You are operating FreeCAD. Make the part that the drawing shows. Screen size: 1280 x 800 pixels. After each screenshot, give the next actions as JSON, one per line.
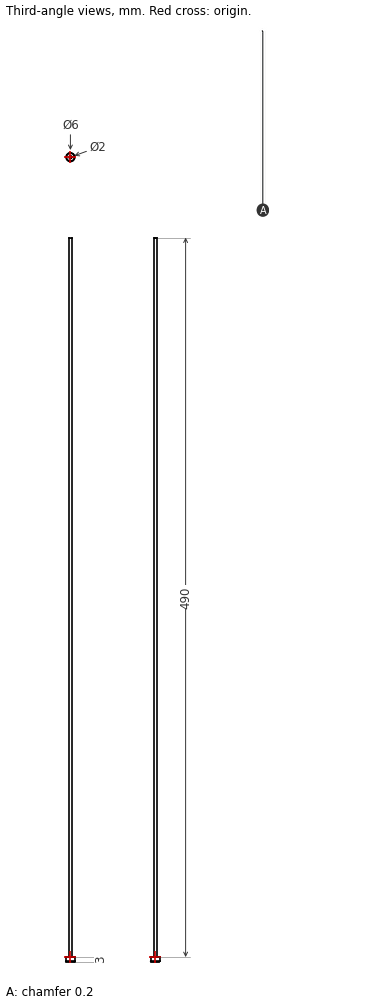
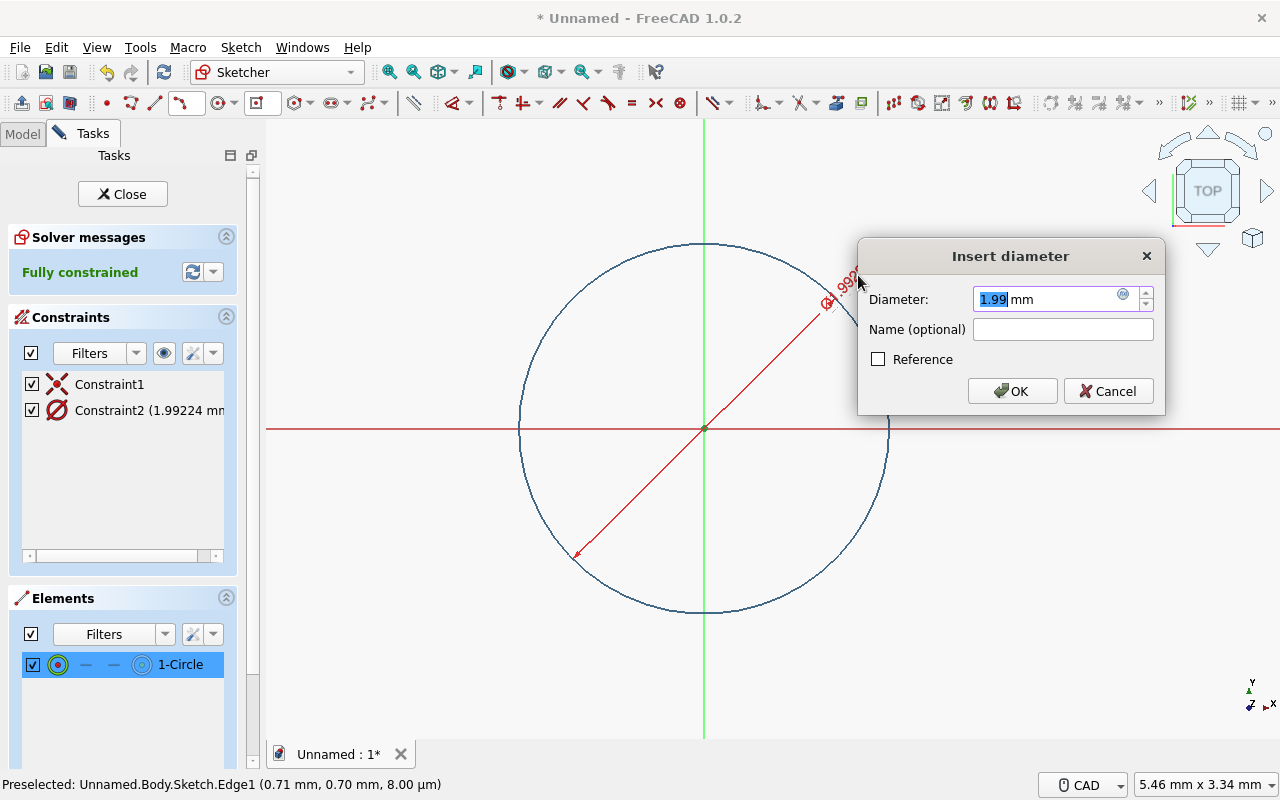
{"action": "type", "text": "2"}
{"action": "key", "text": "Return"}
{"action": "key", "text": "Escape"}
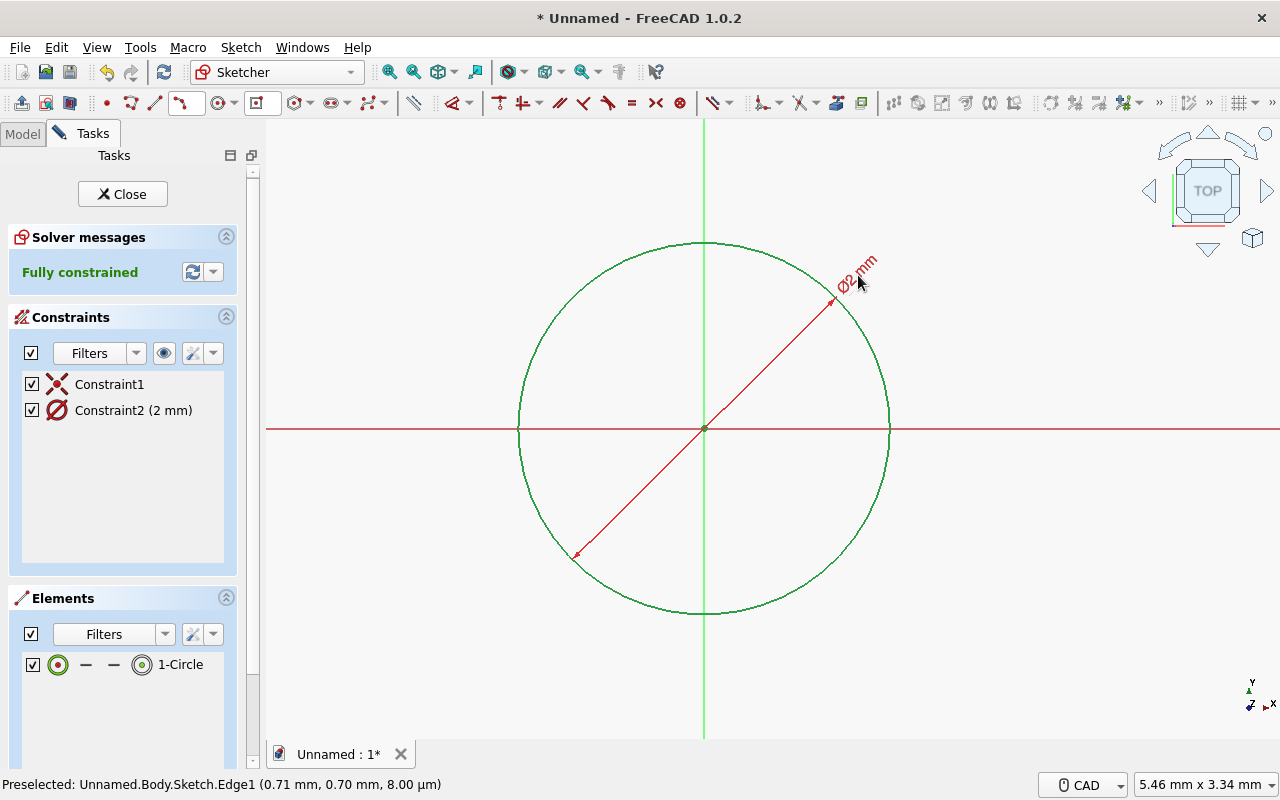
{"action": "left_click", "coordinate": [123, 194]}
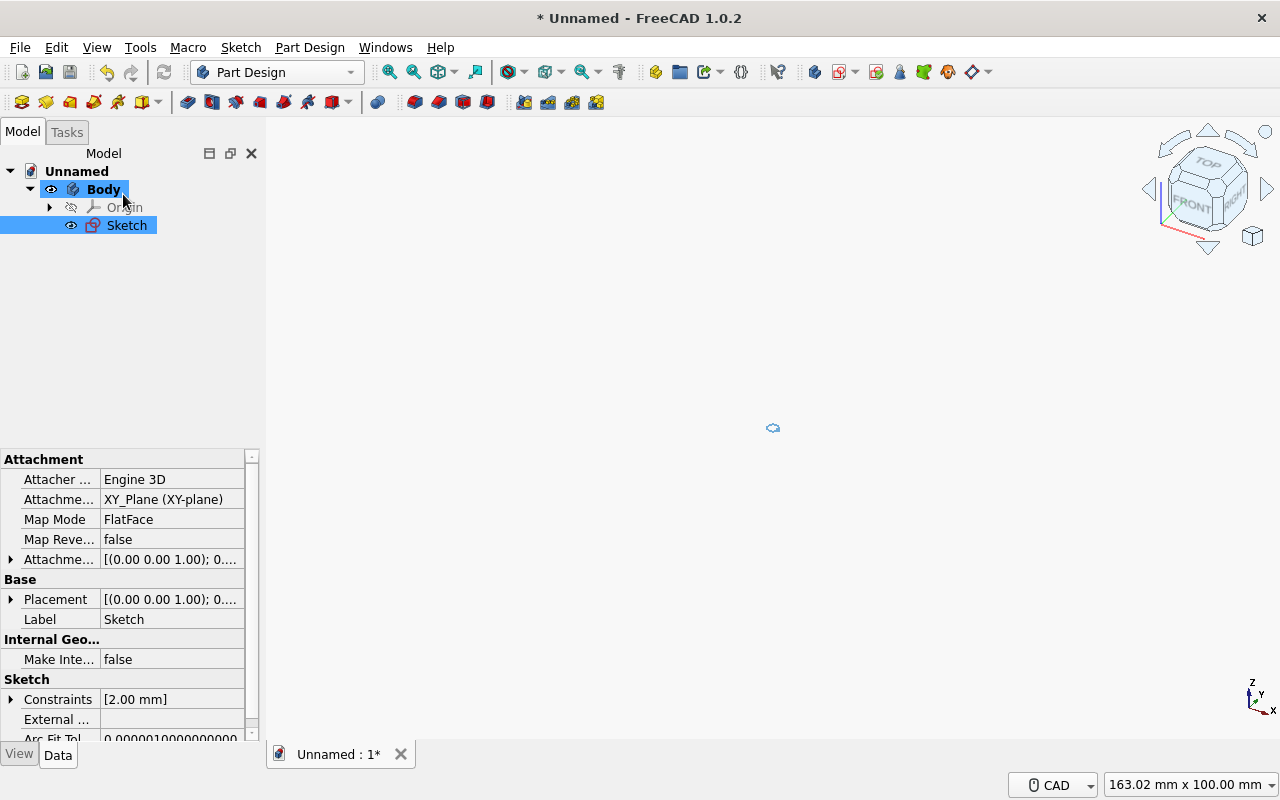
{"action": "left_click", "coordinate": [22, 102]}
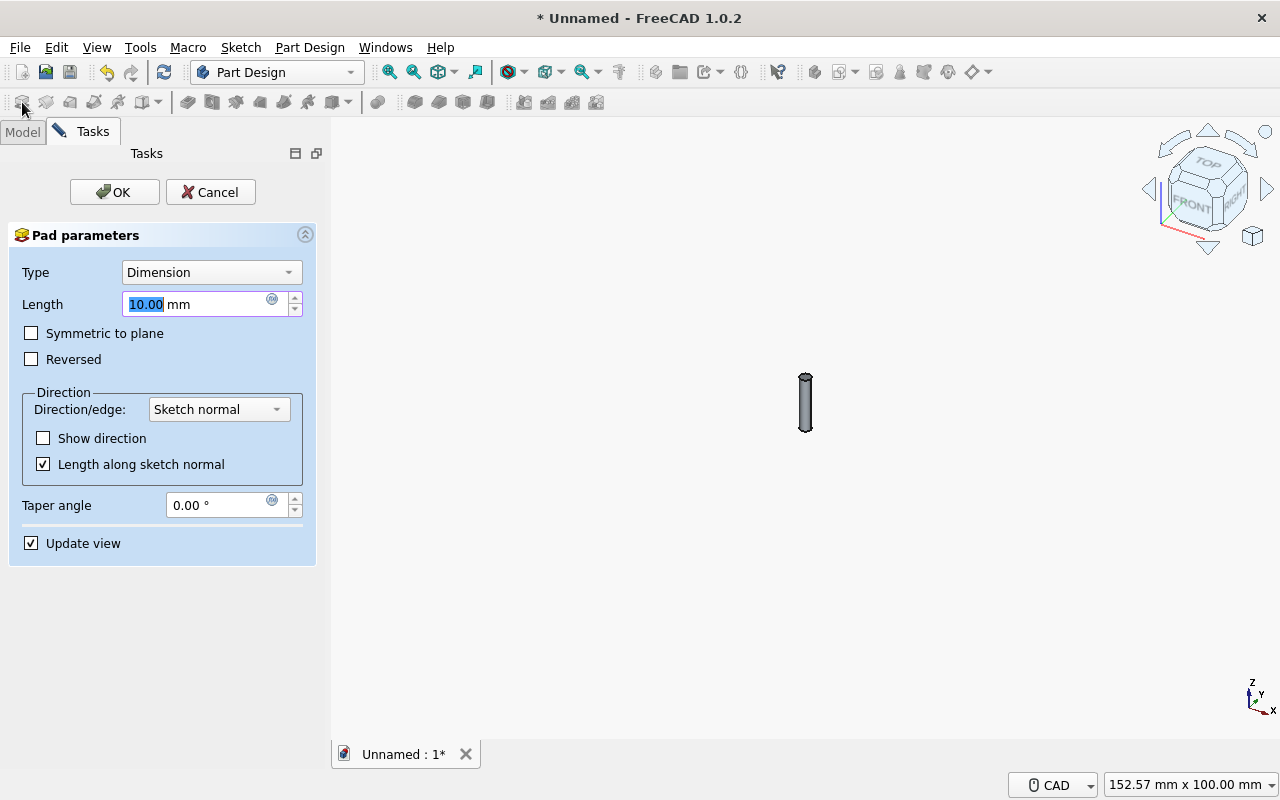
{"action": "type", "text": "490"}
{"action": "key", "text": "Tab"}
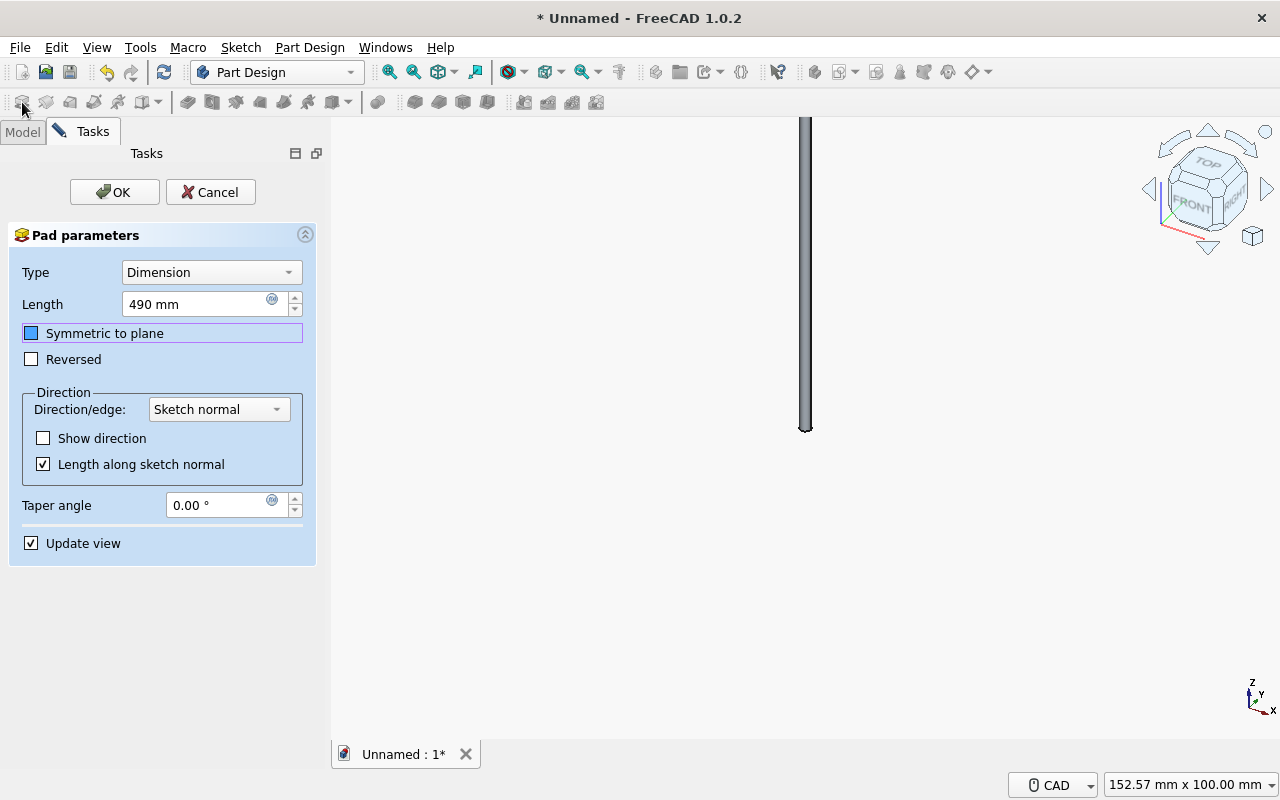
{"action": "left_click", "coordinate": [115, 192]}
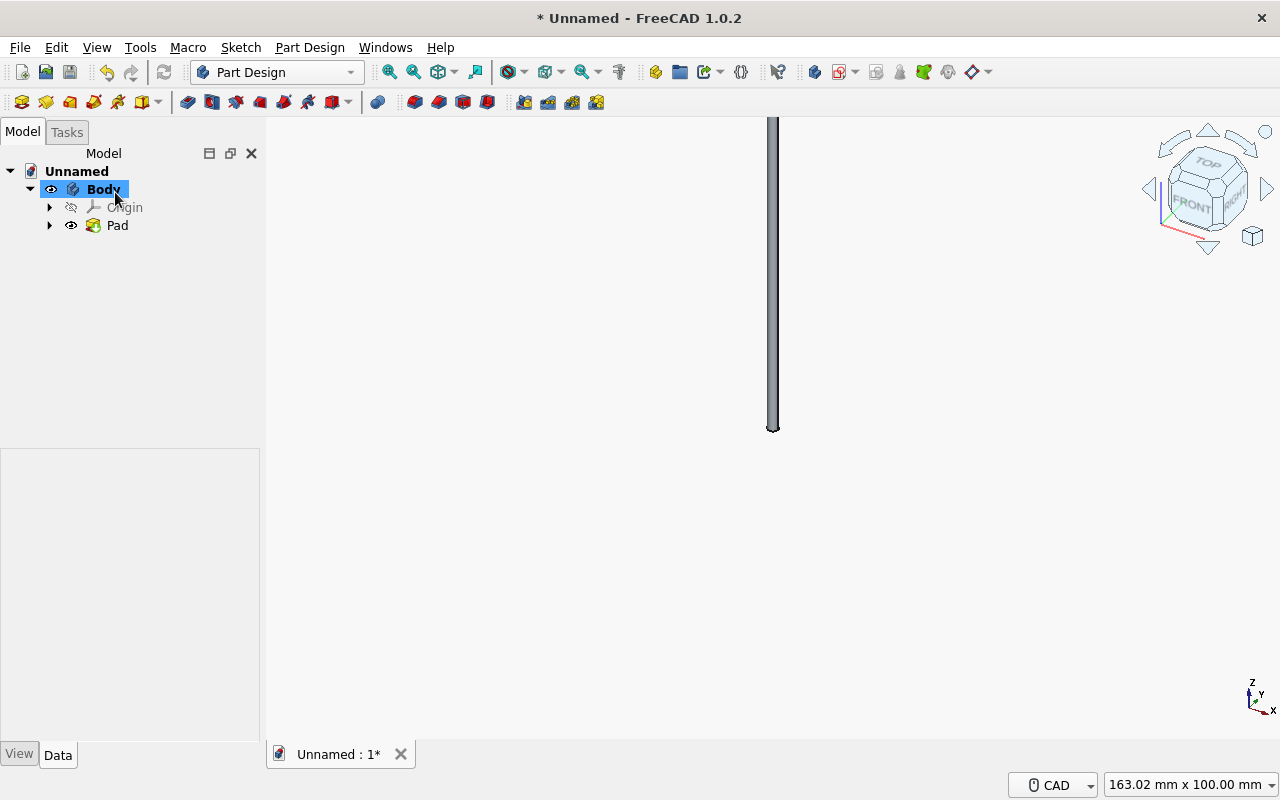
{"action": "key", "text": "v f"}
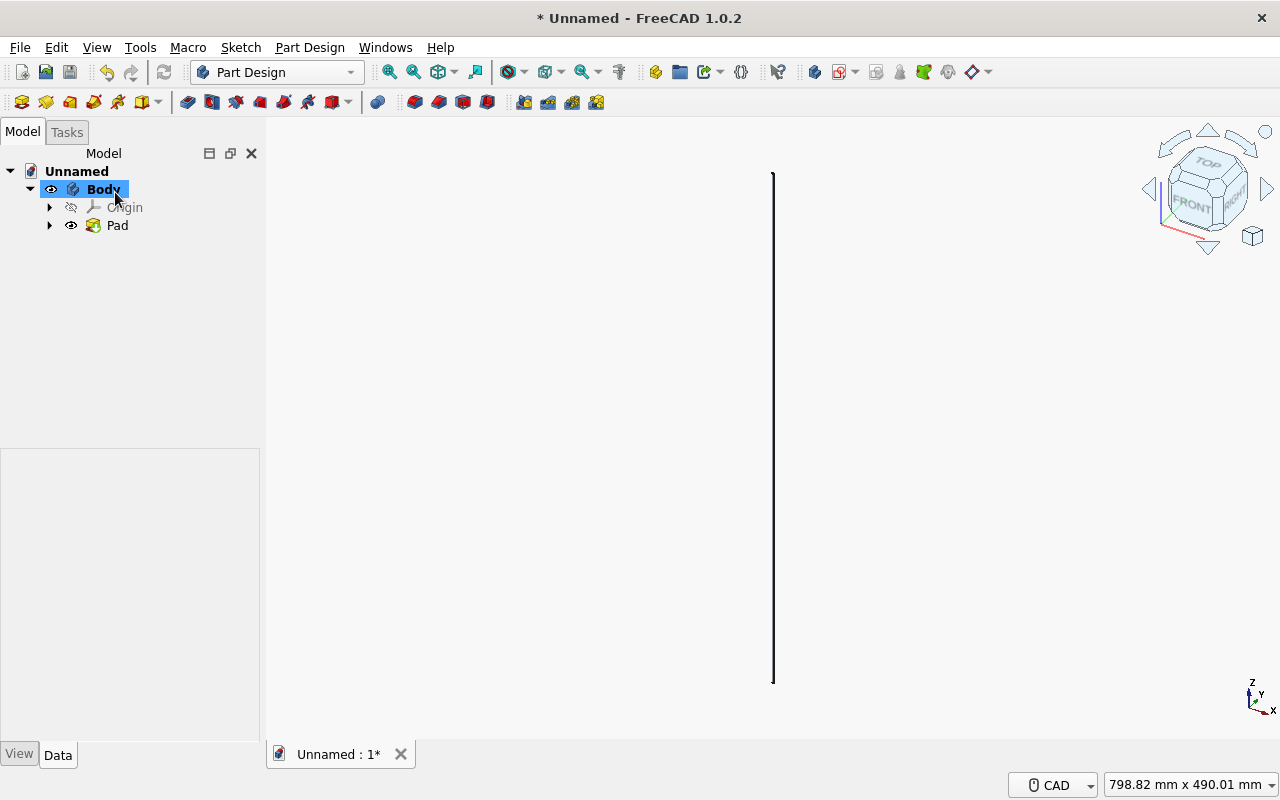
{"action": "key", "text": "5"}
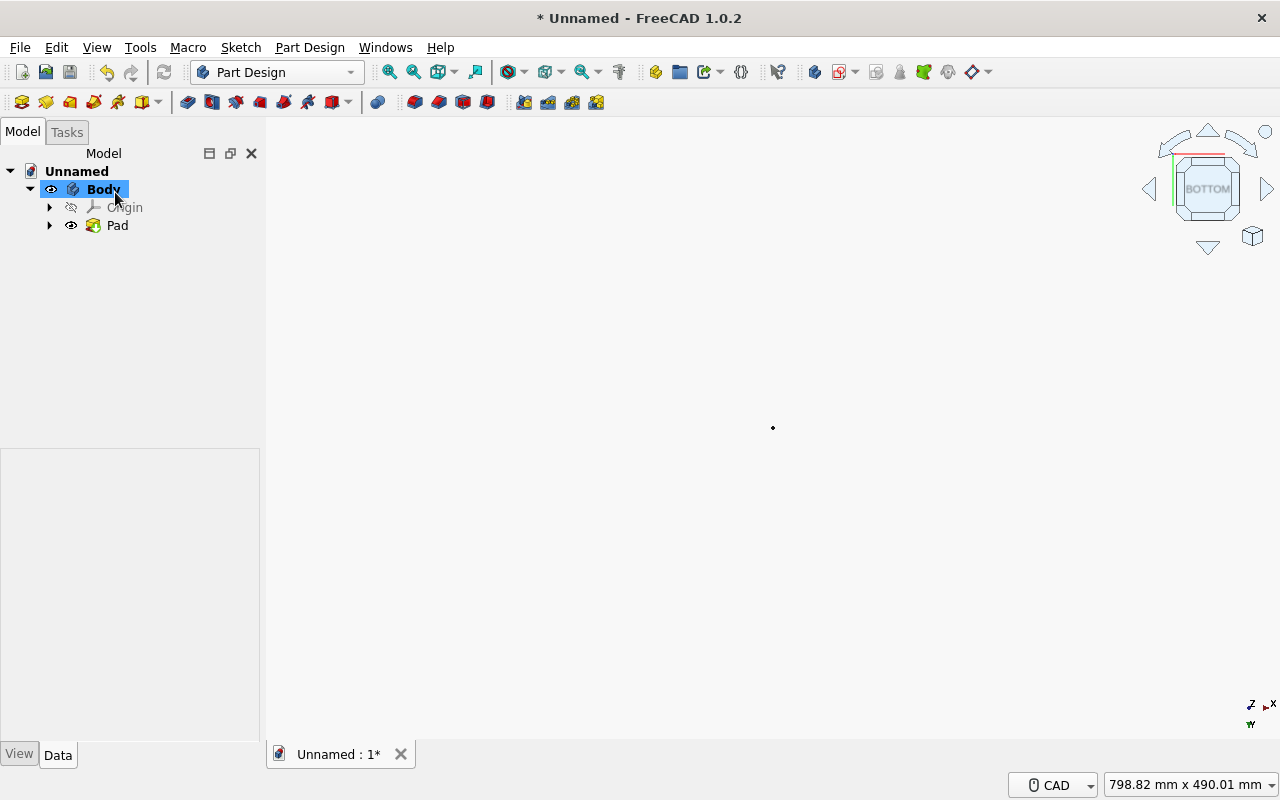
{"action": "key", "text": "v f"}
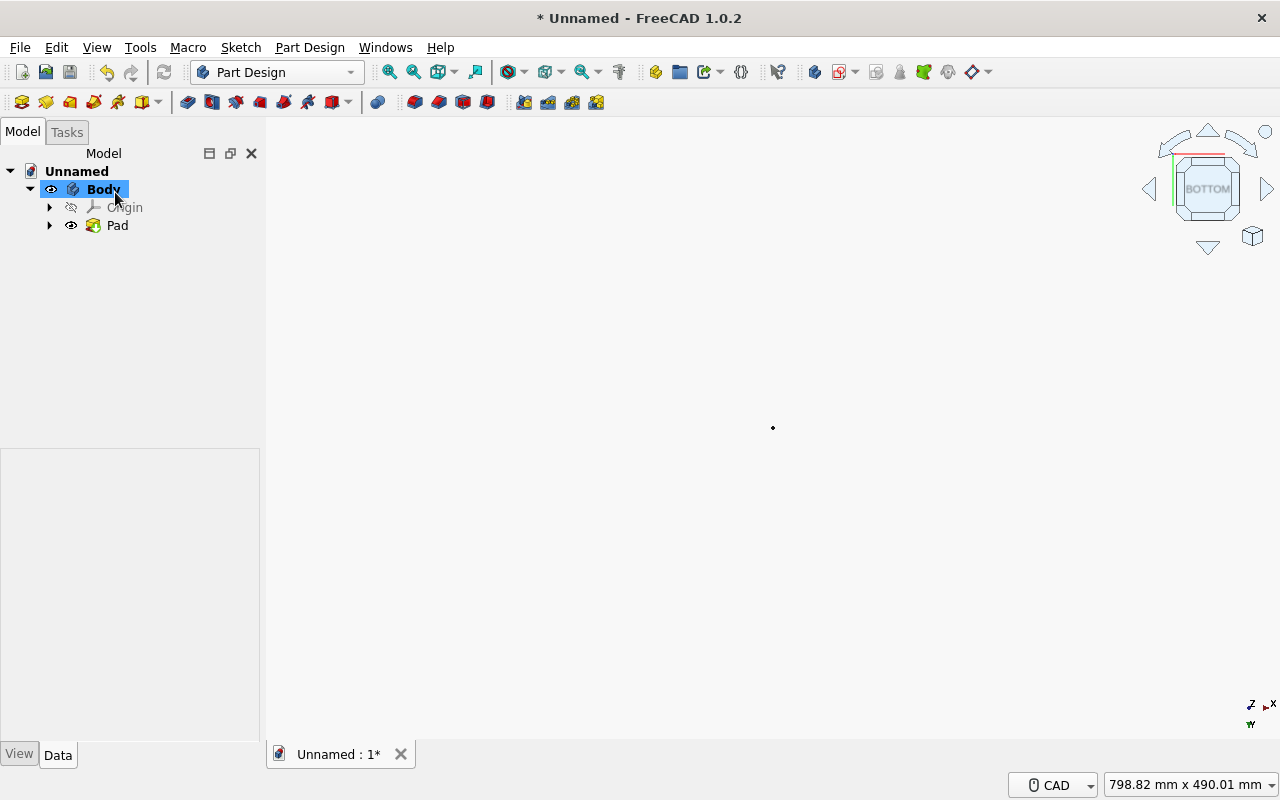
{"action": "scroll", "coordinate": [773, 427], "scroll_direction": "up", "scroll_amount": 12}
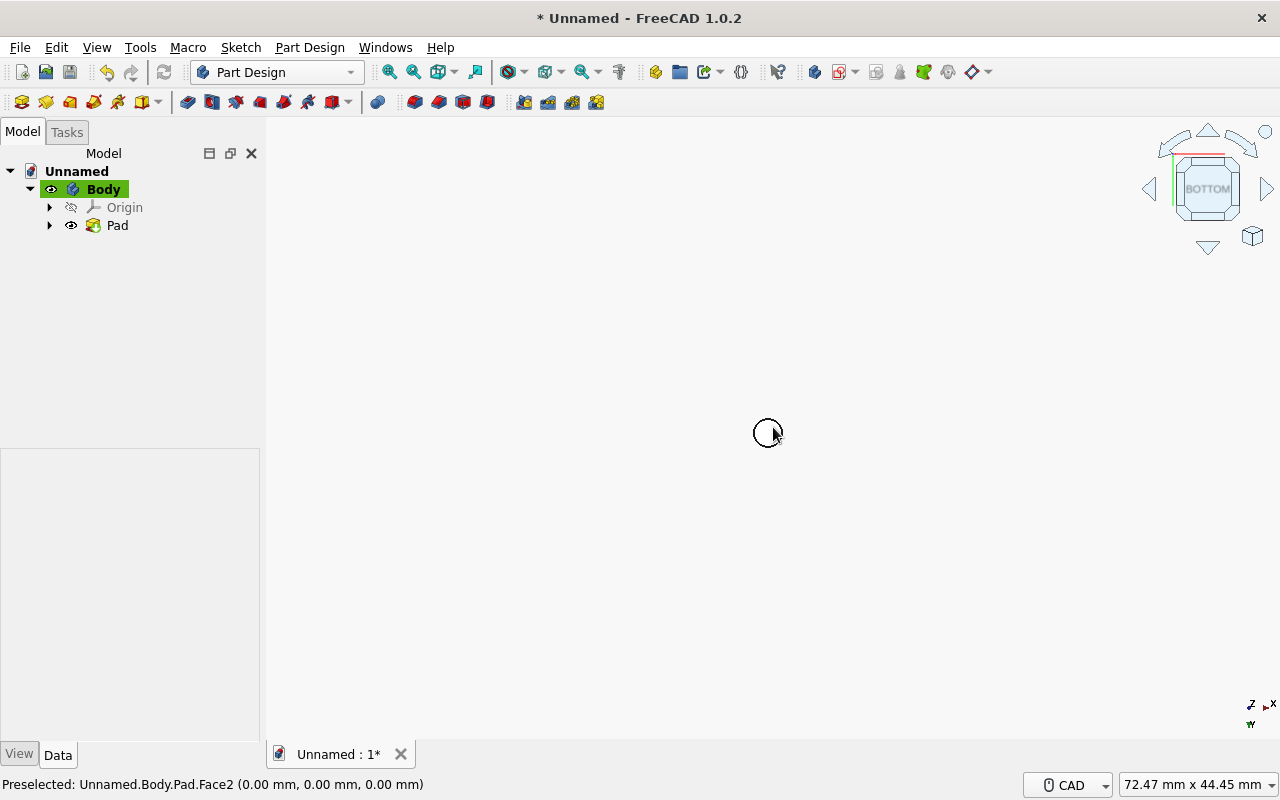
{"action": "left_click", "coordinate": [768, 432]}